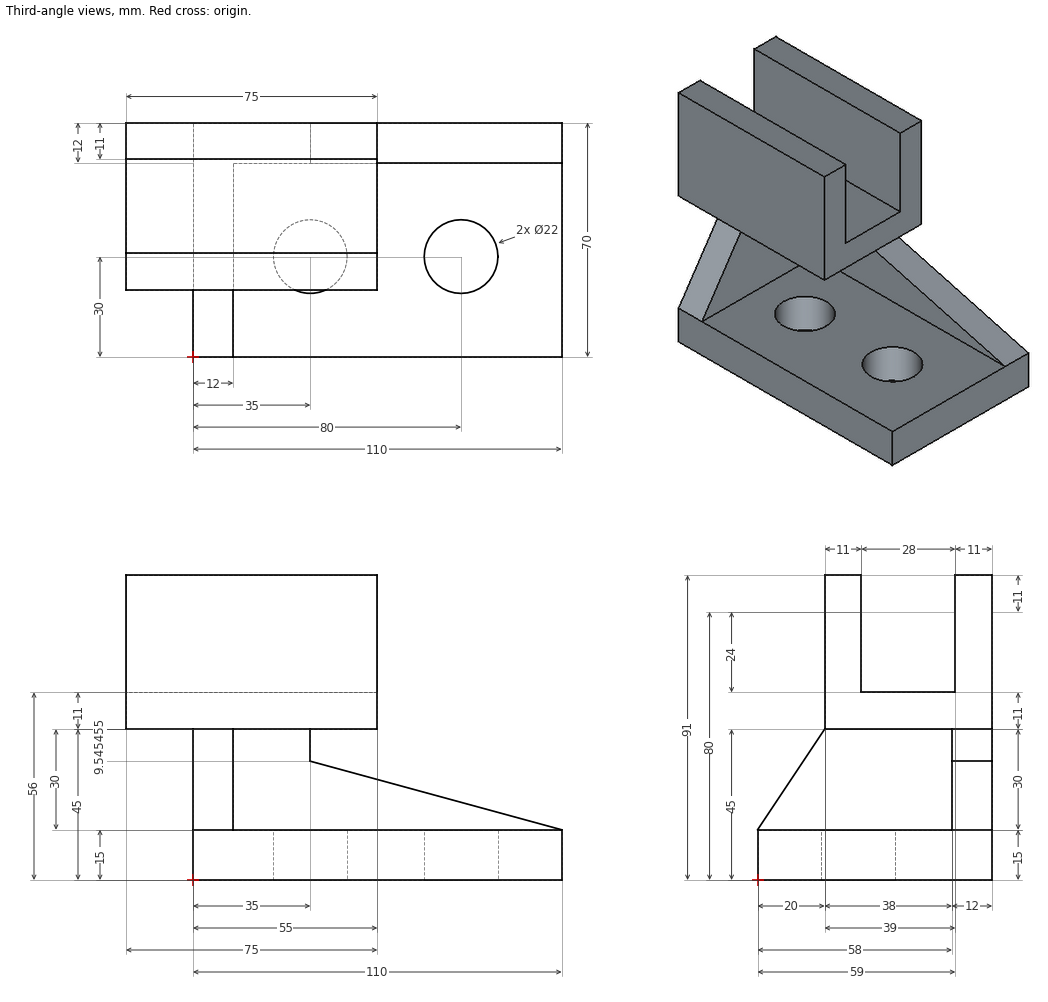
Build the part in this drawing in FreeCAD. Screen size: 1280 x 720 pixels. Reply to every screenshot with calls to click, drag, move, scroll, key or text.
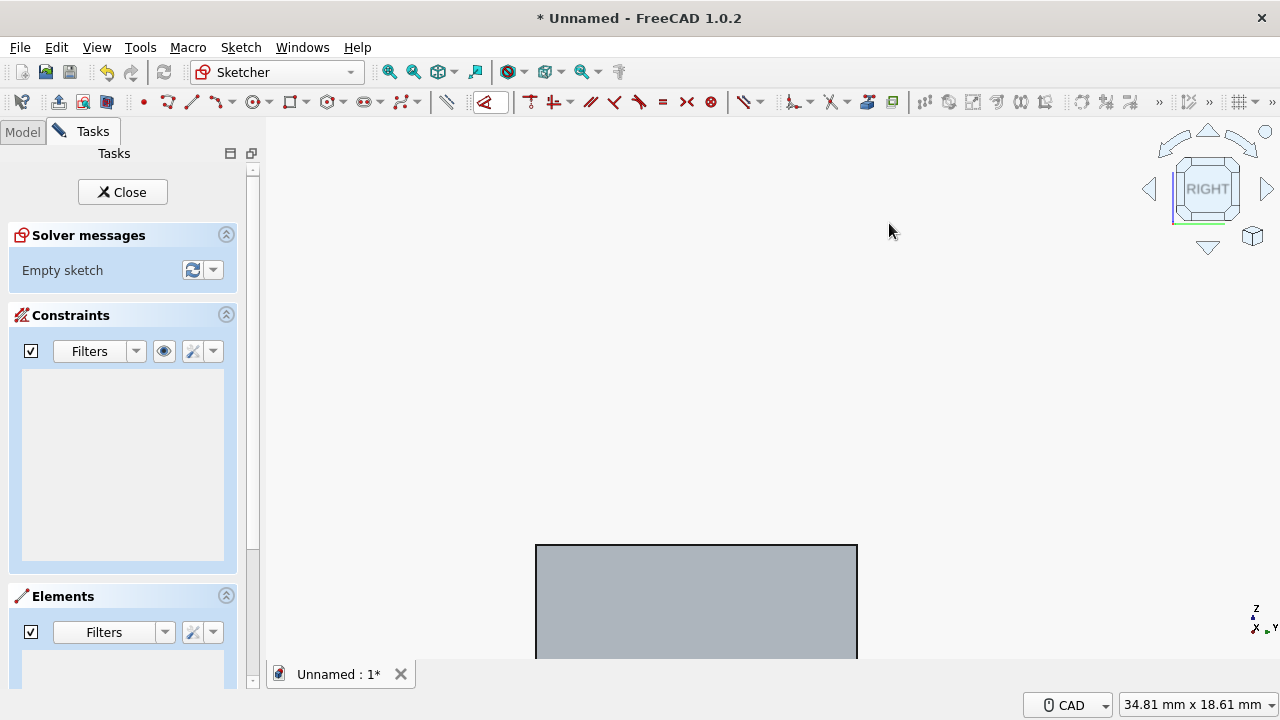
click(290, 102)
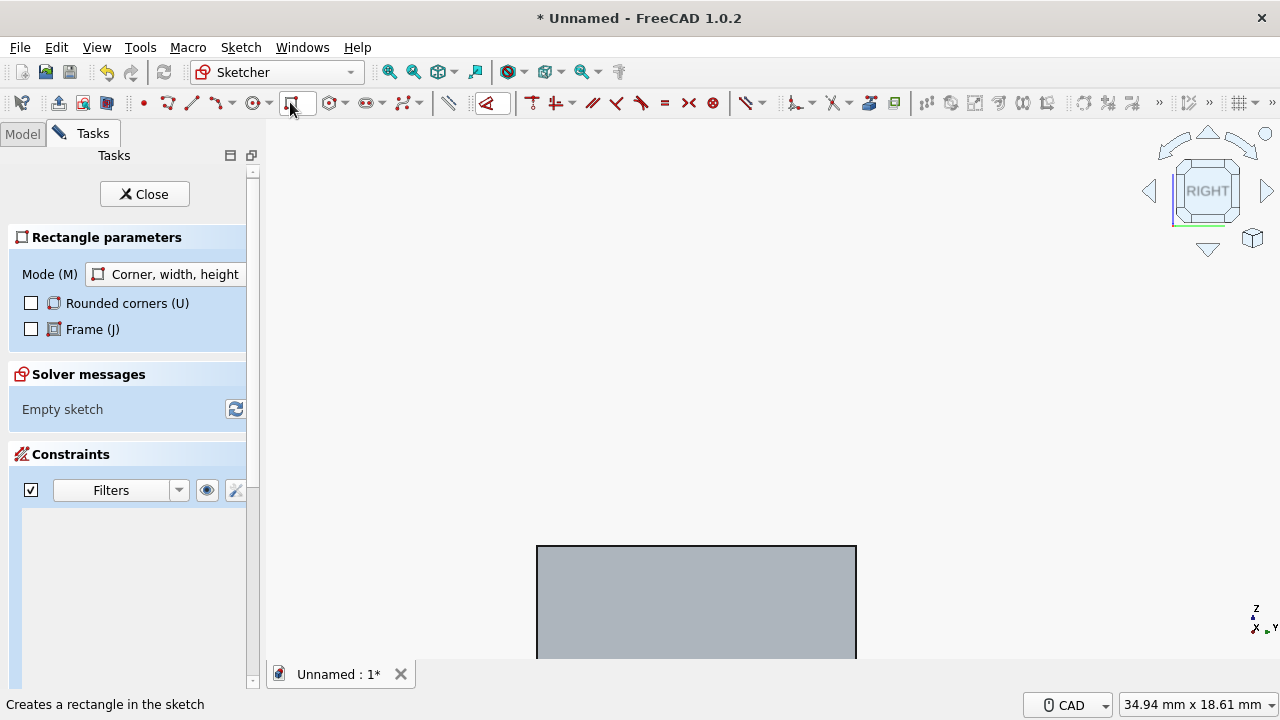
click(537, 227)
move(856, 546)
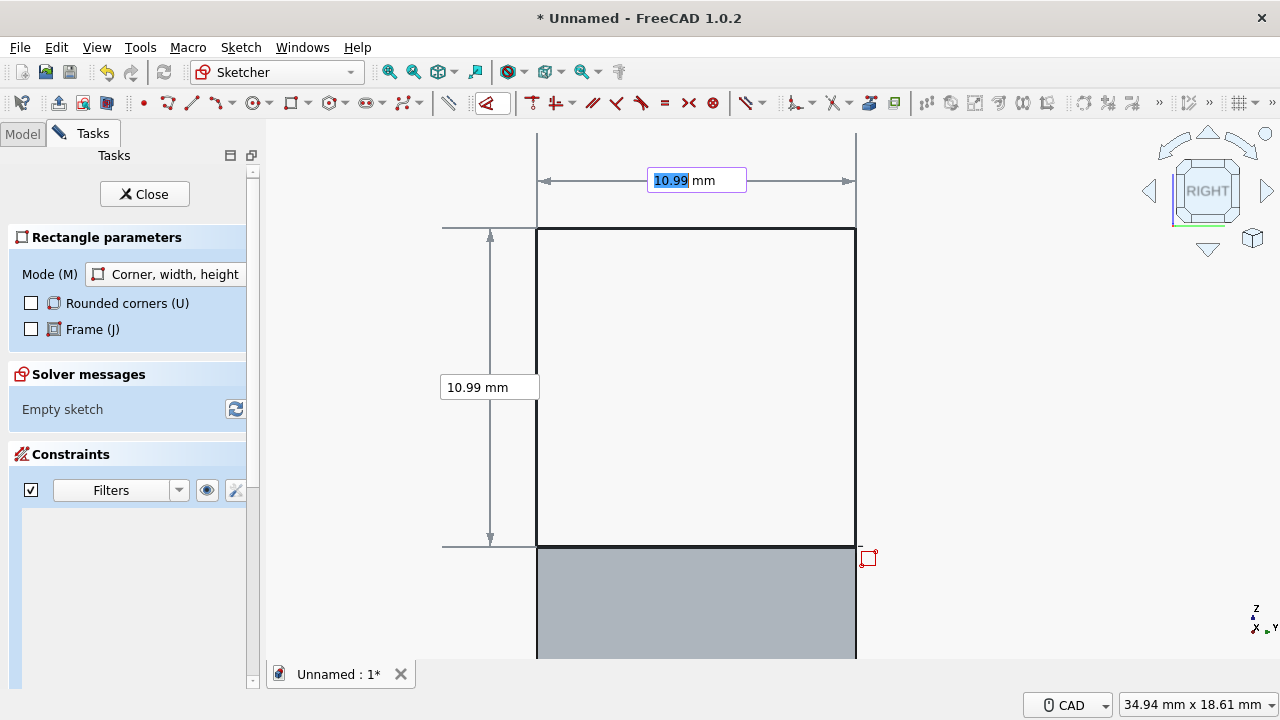
text(11)
key(Tab)
text(11)
key(Return)
key(Escape)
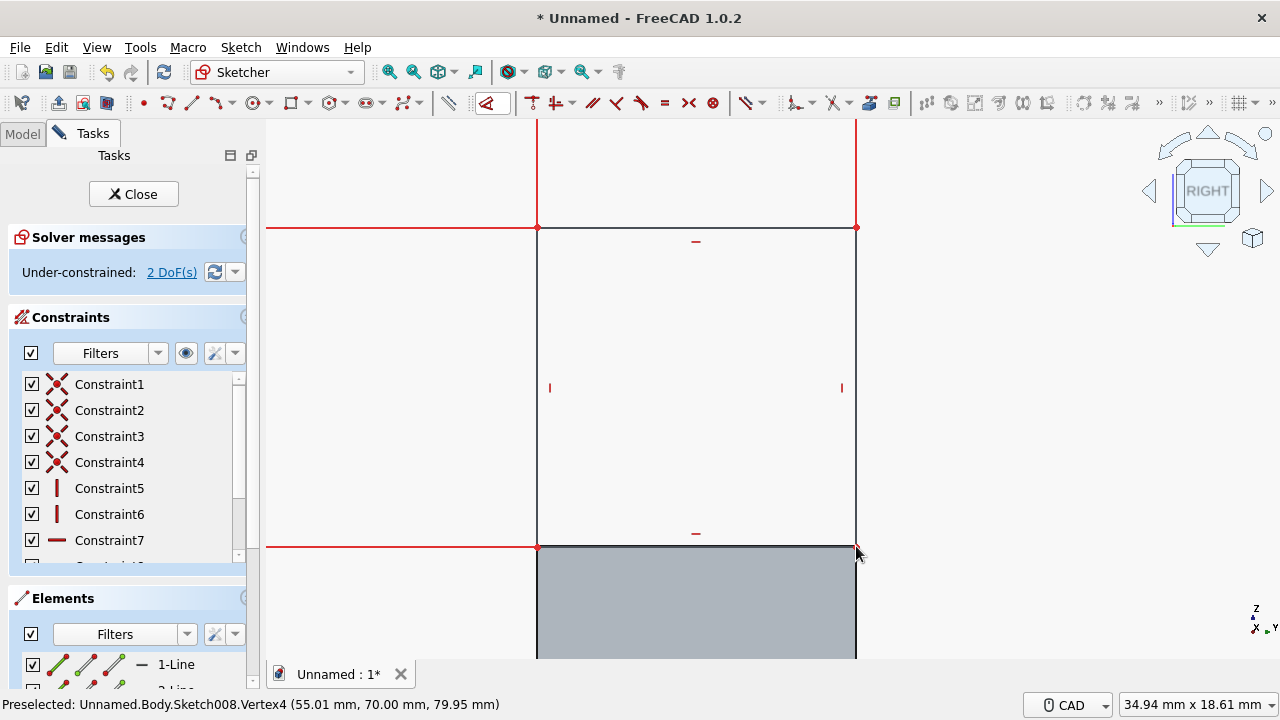
click(537, 228)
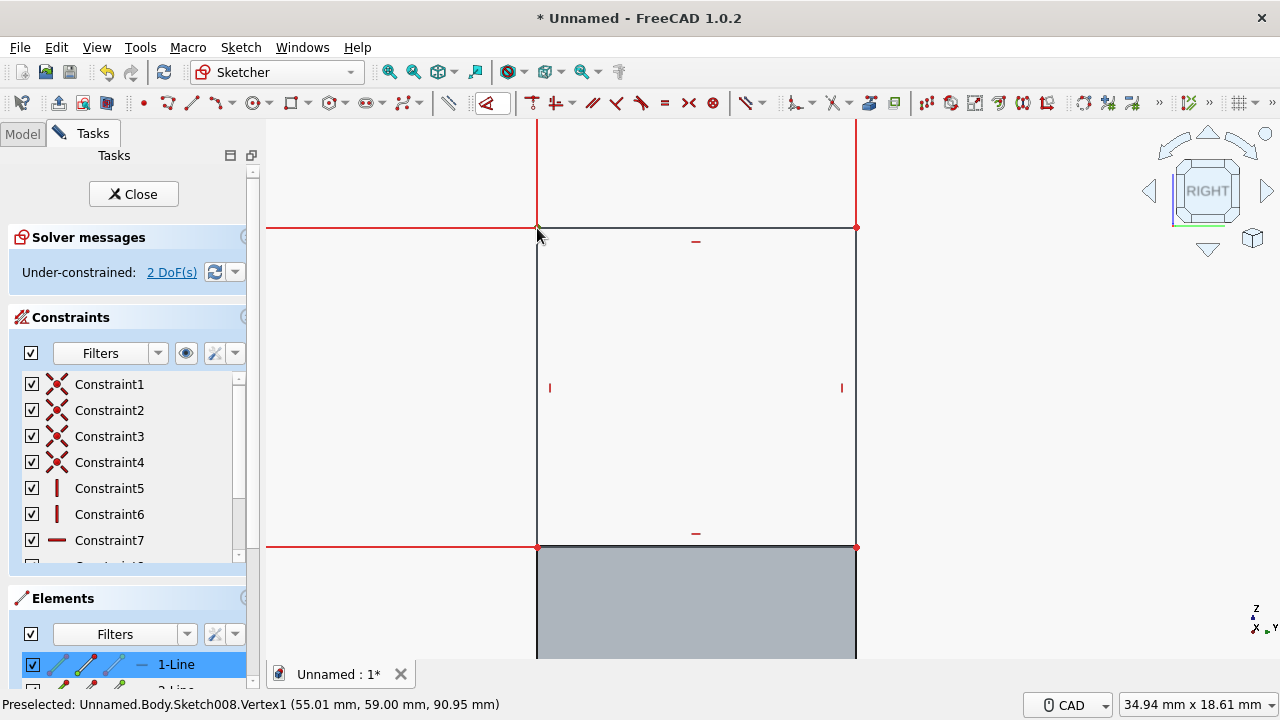
key(l)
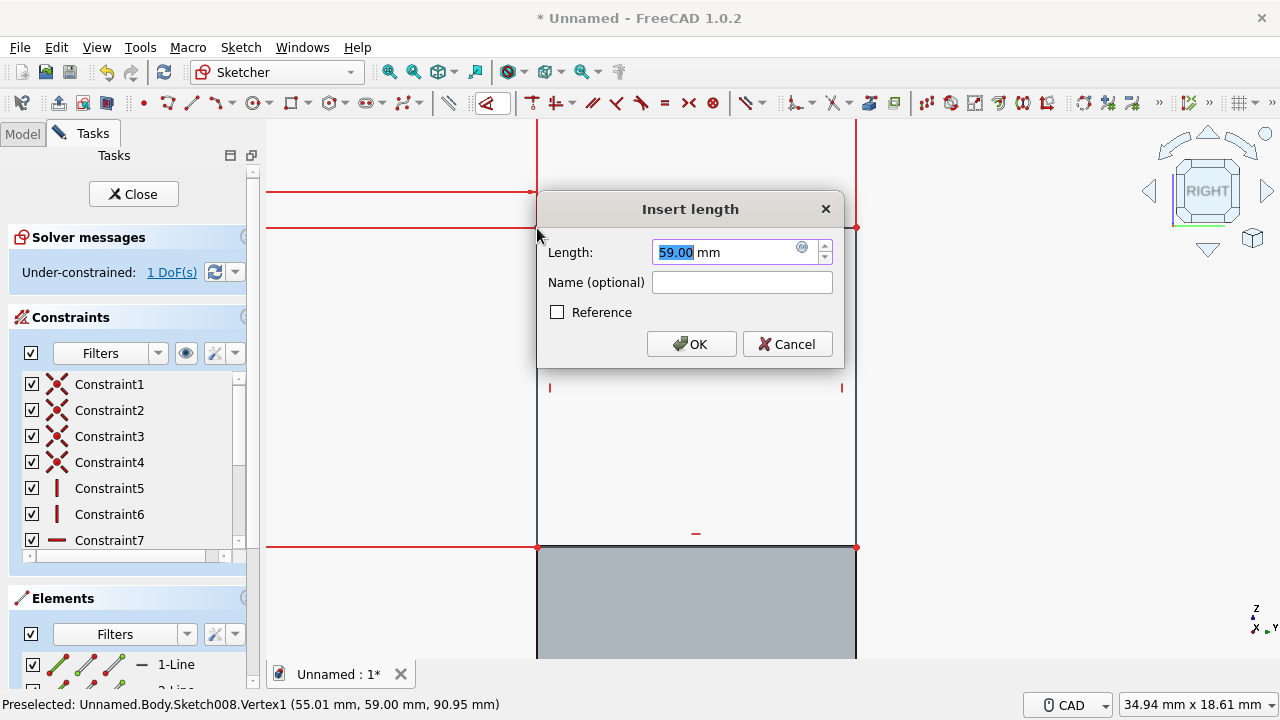
text(59)
key(Return)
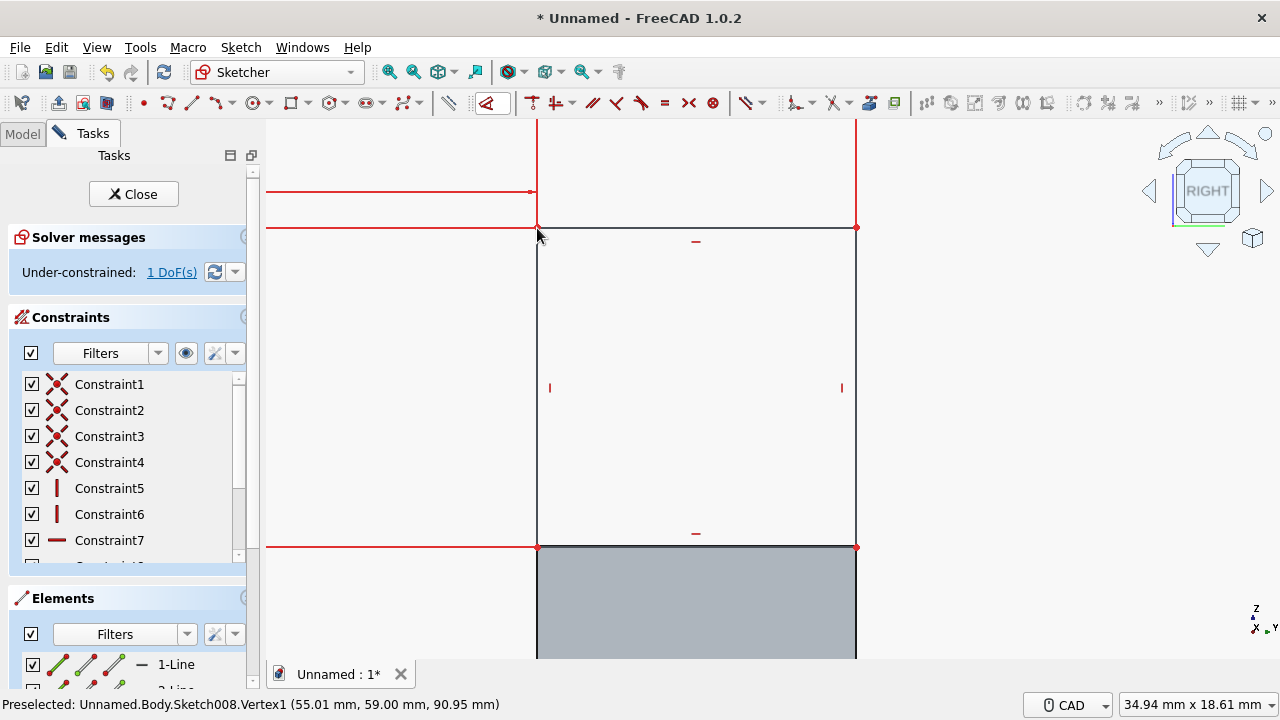
click(537, 228)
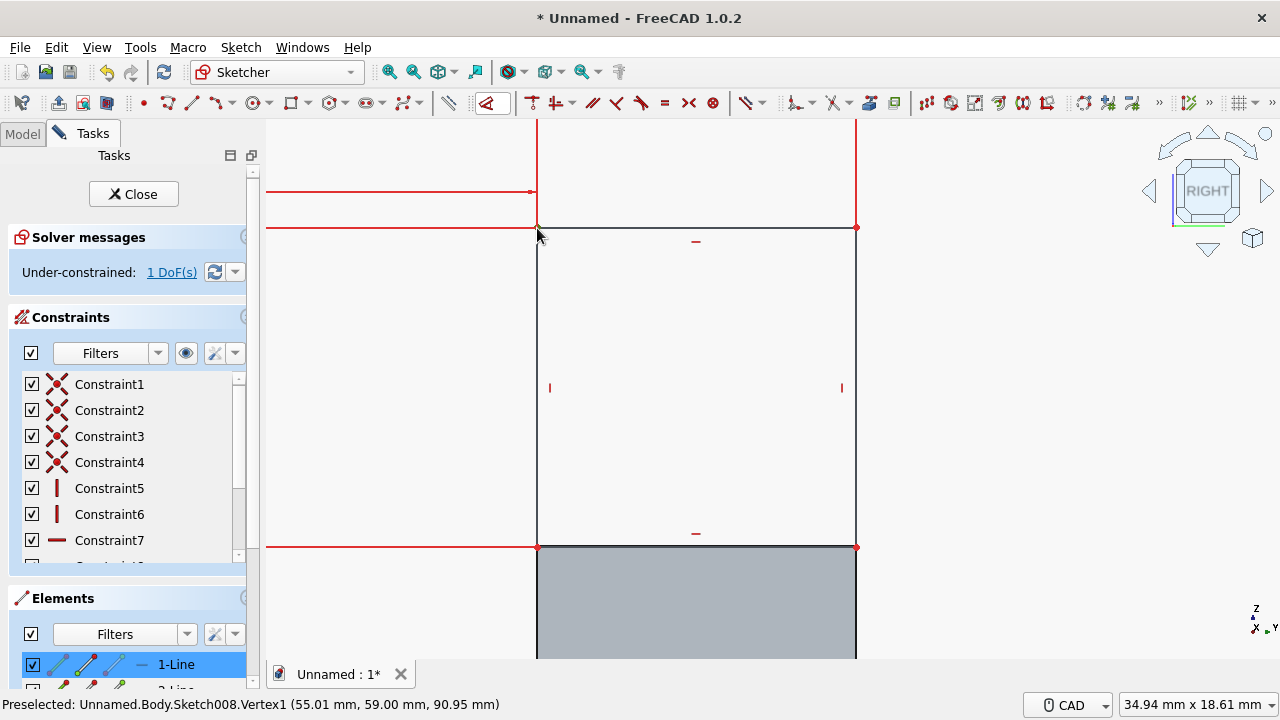
key(i)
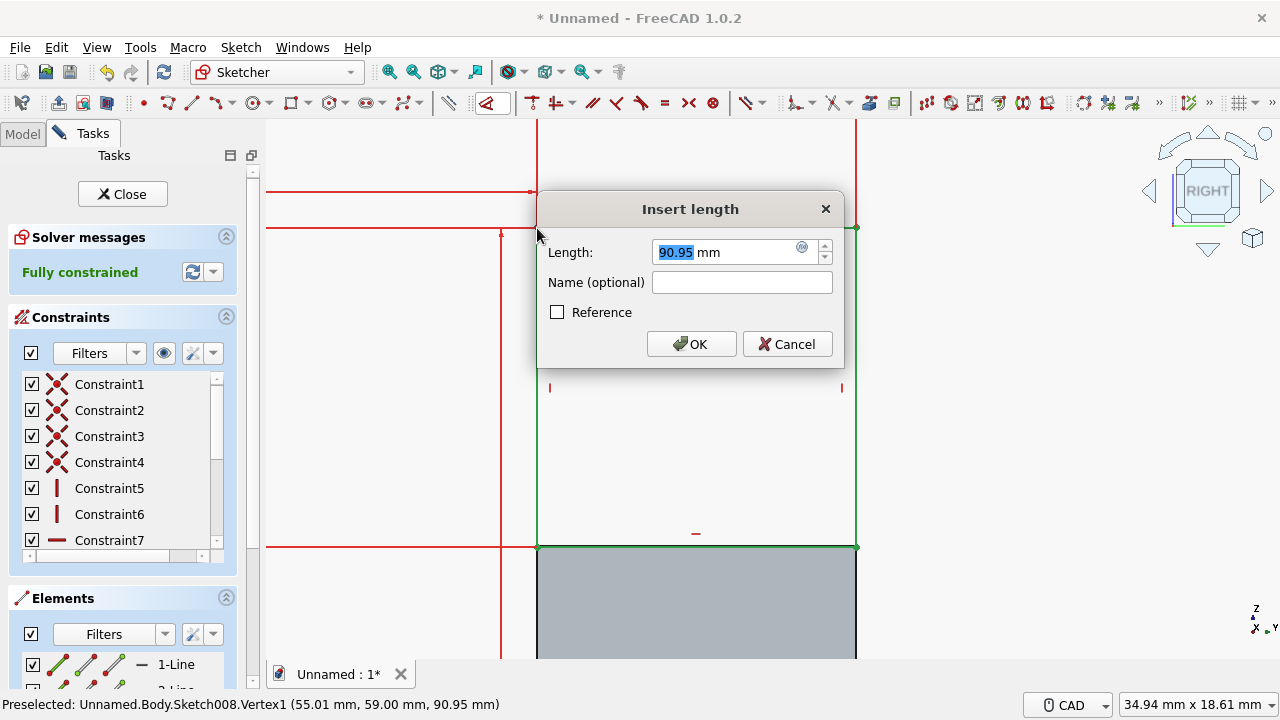
text(91)
key(Return)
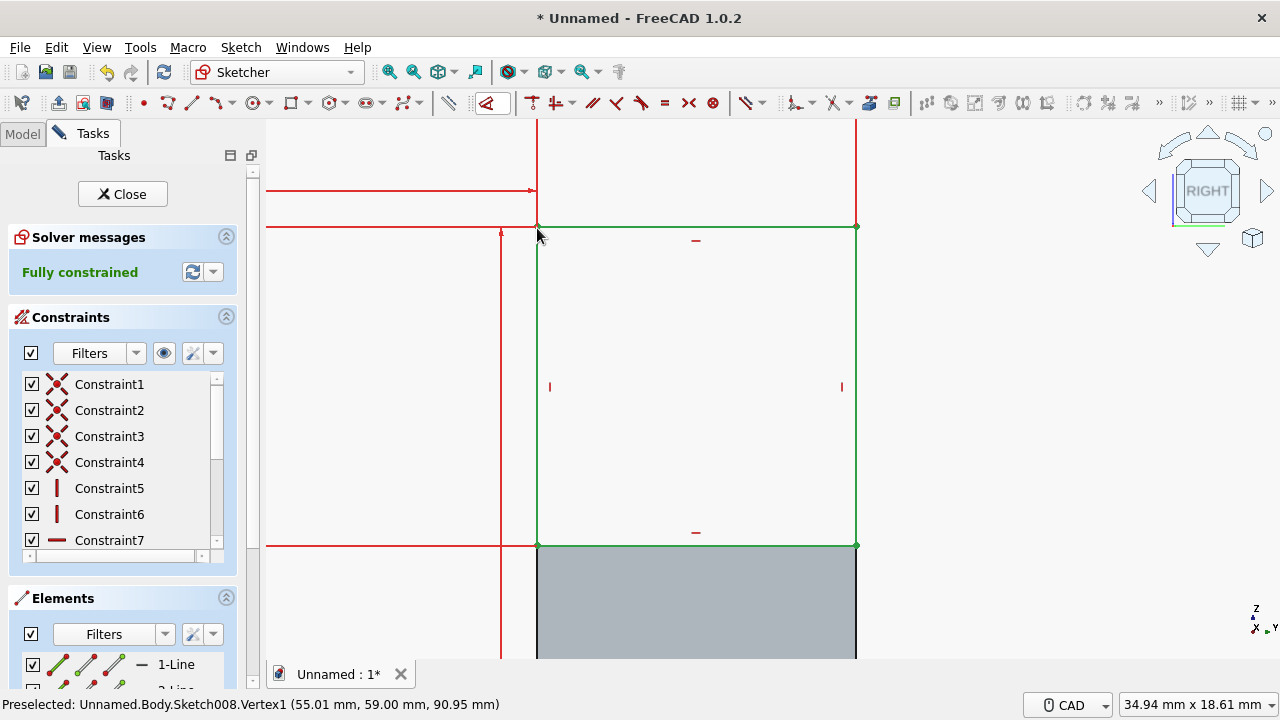
click(123, 194)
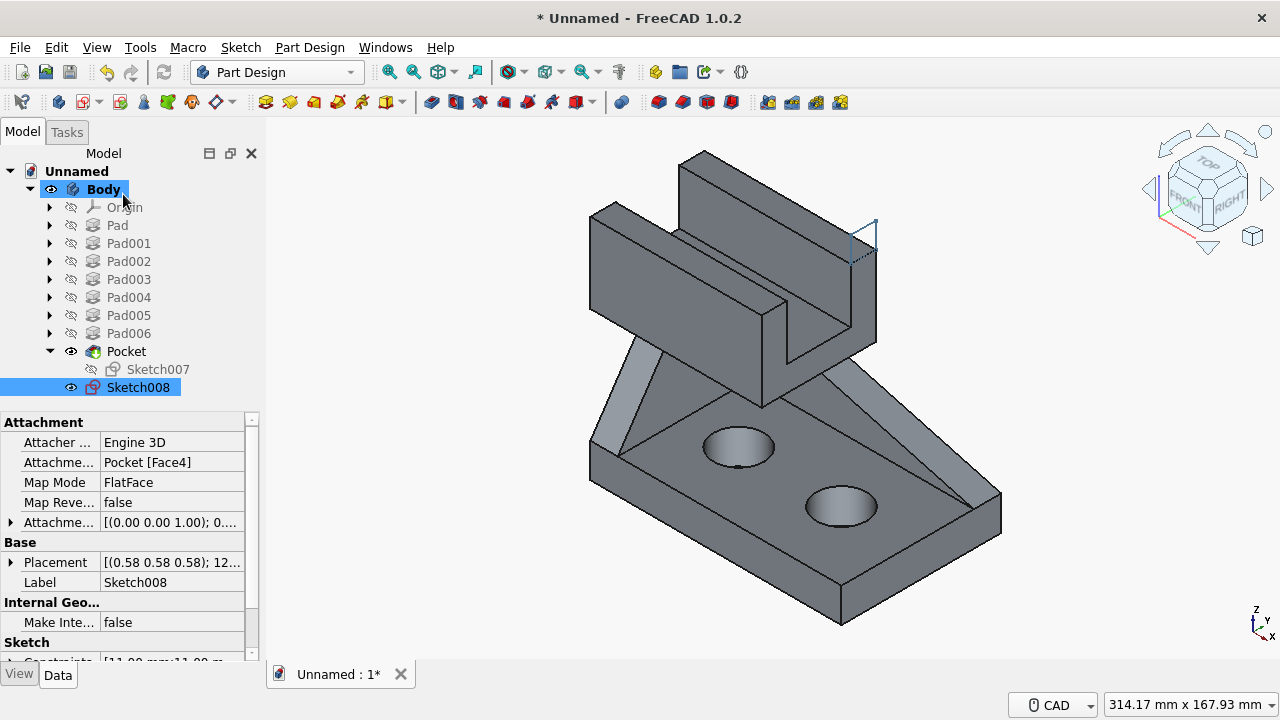
click(266, 102)